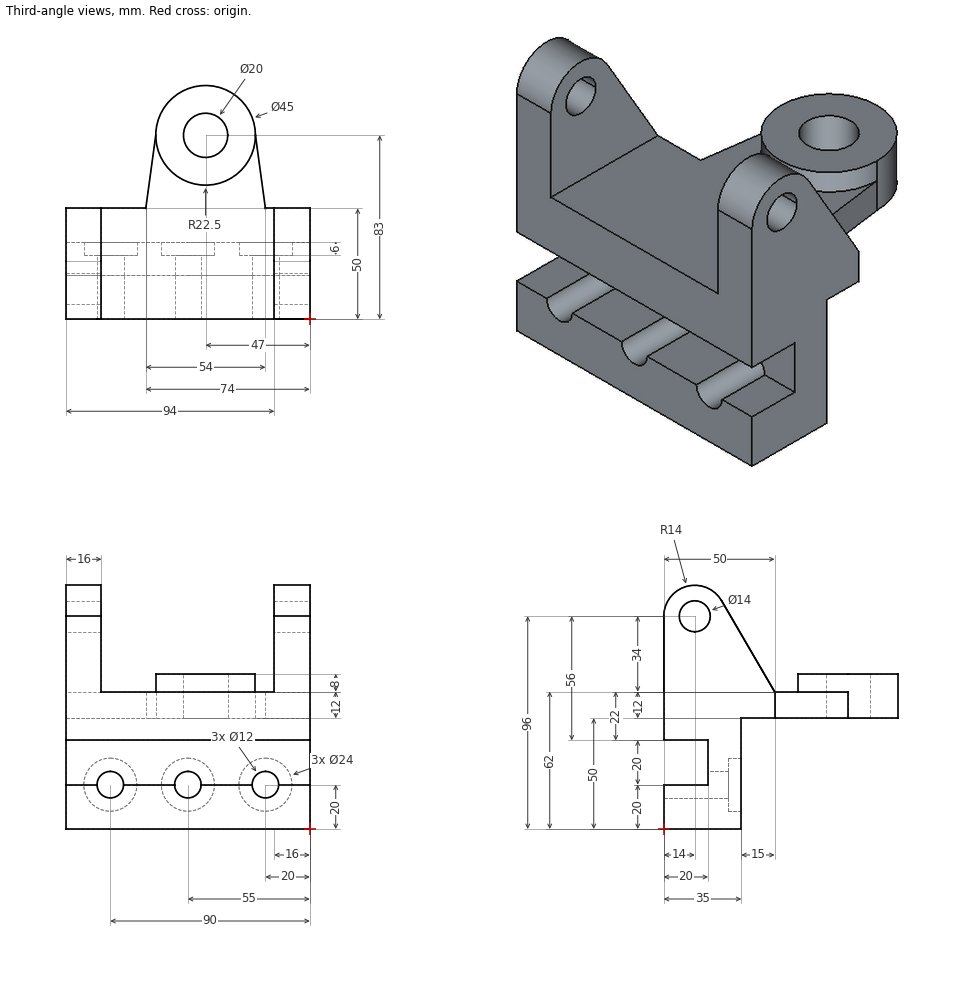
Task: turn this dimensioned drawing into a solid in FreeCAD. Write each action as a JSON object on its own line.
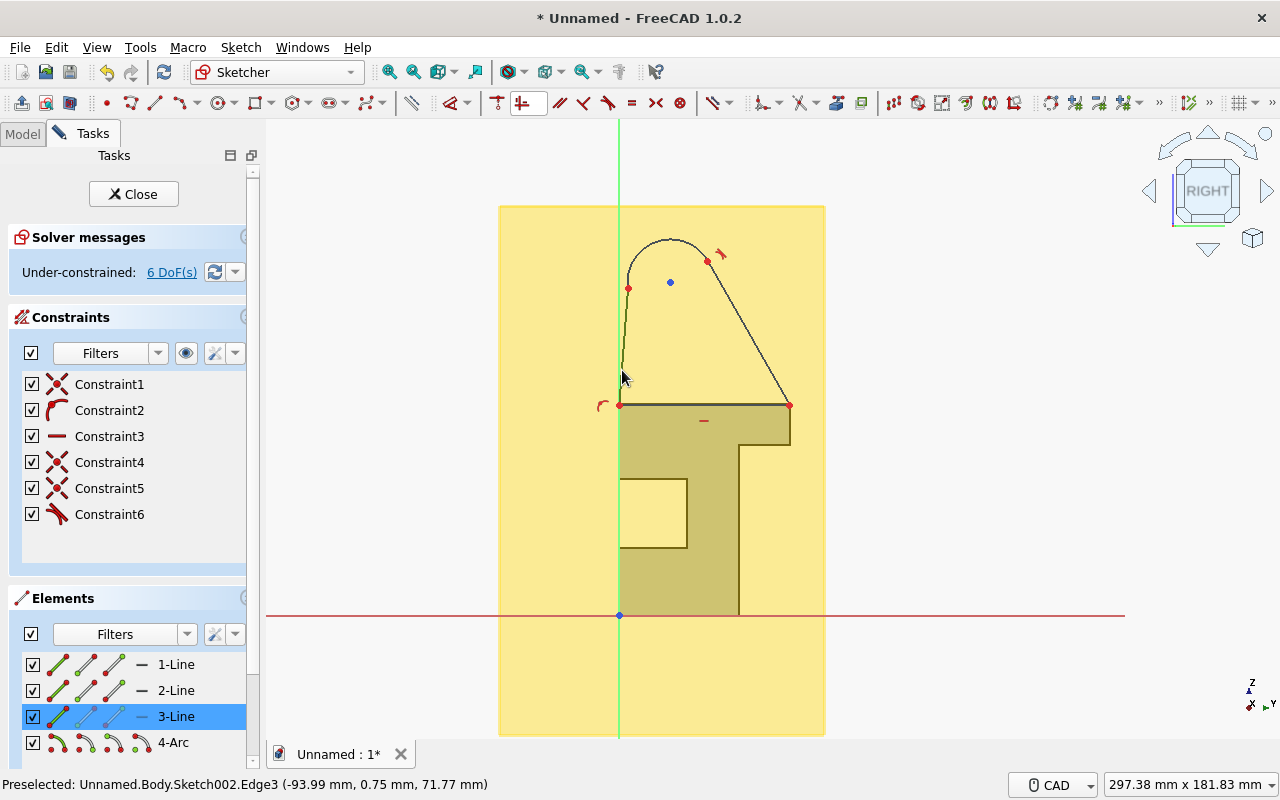
{"action": "left_click", "coordinate": [680, 241]}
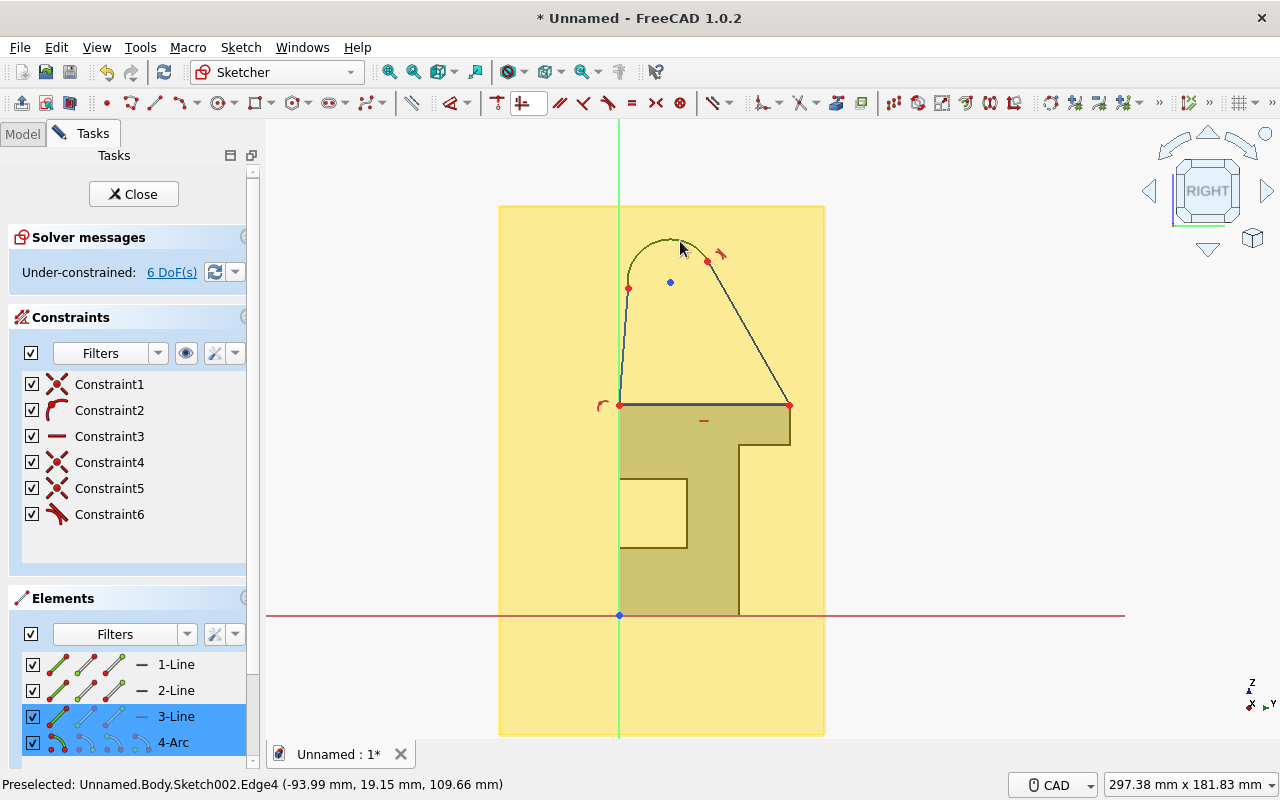
{"action": "left_click", "coordinate": [608, 104]}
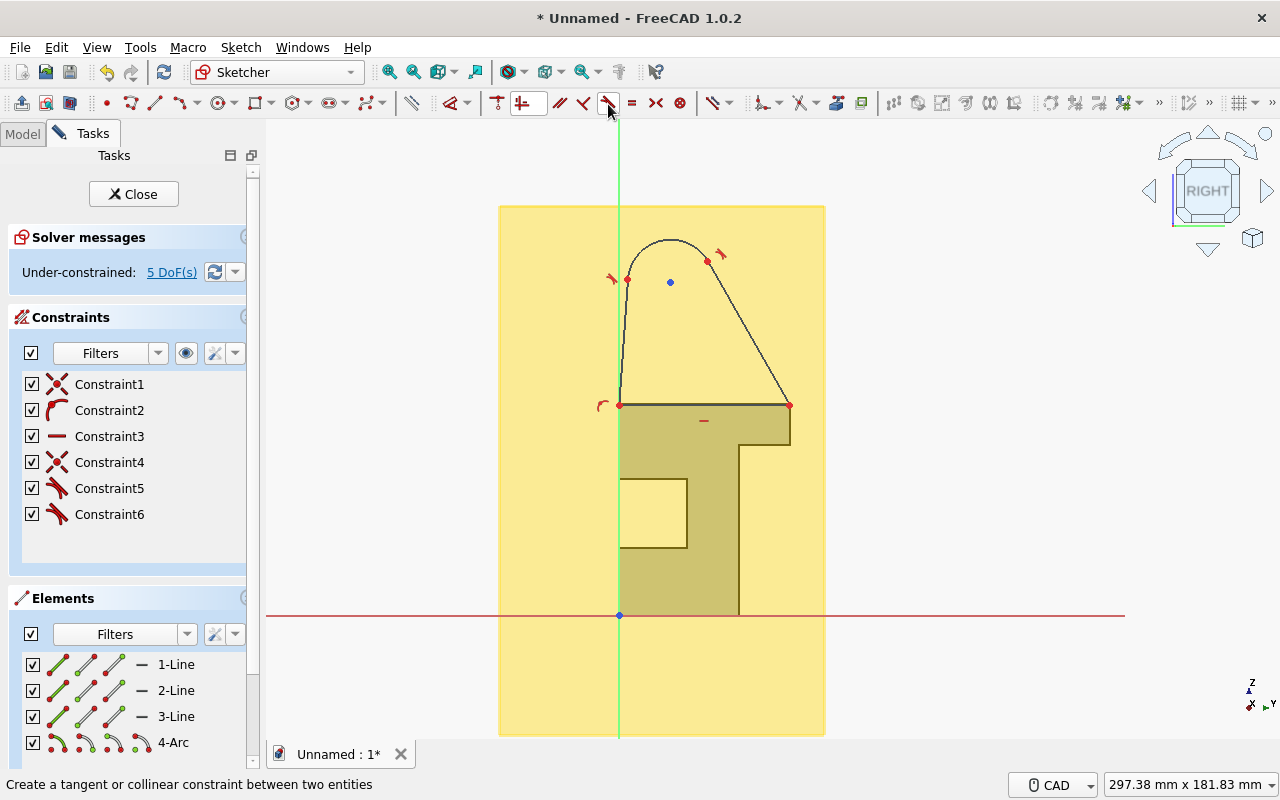
{"action": "left_click", "coordinate": [622, 367]}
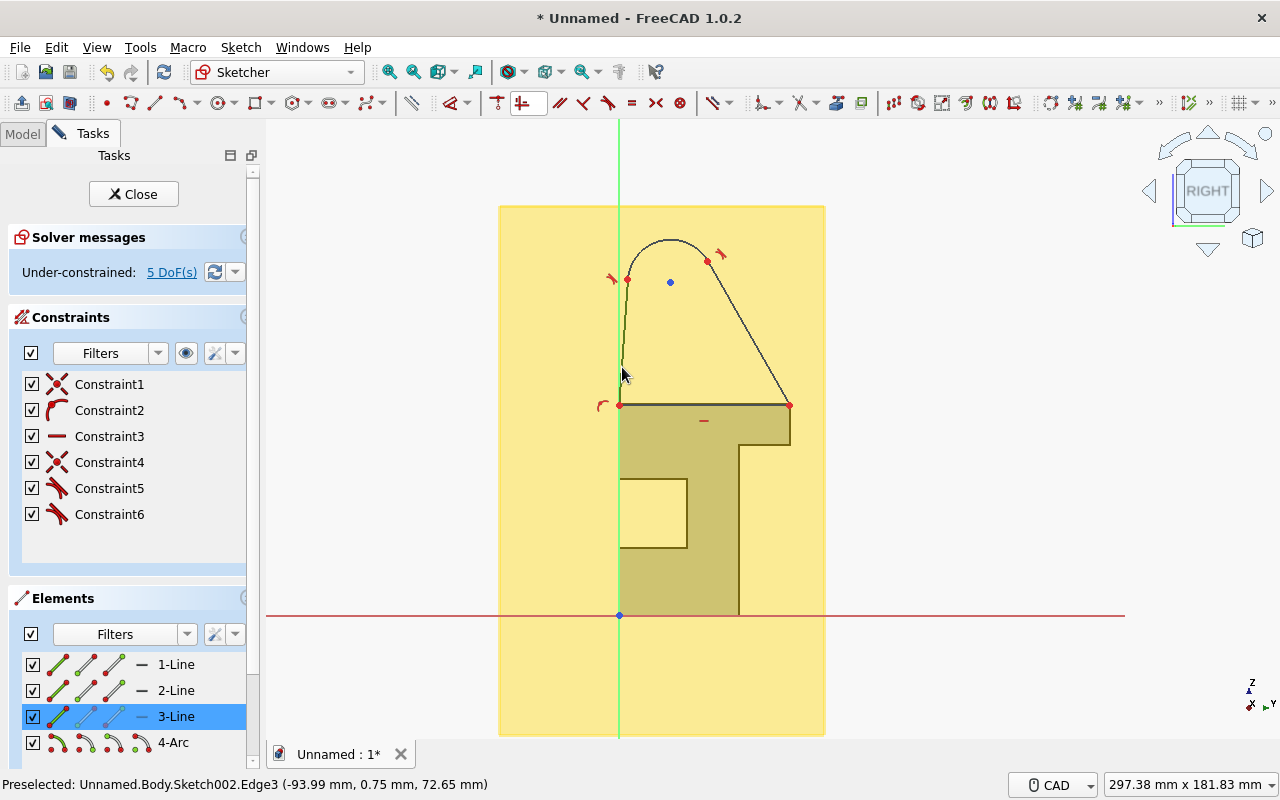
{"action": "left_click", "coordinate": [542, 104]}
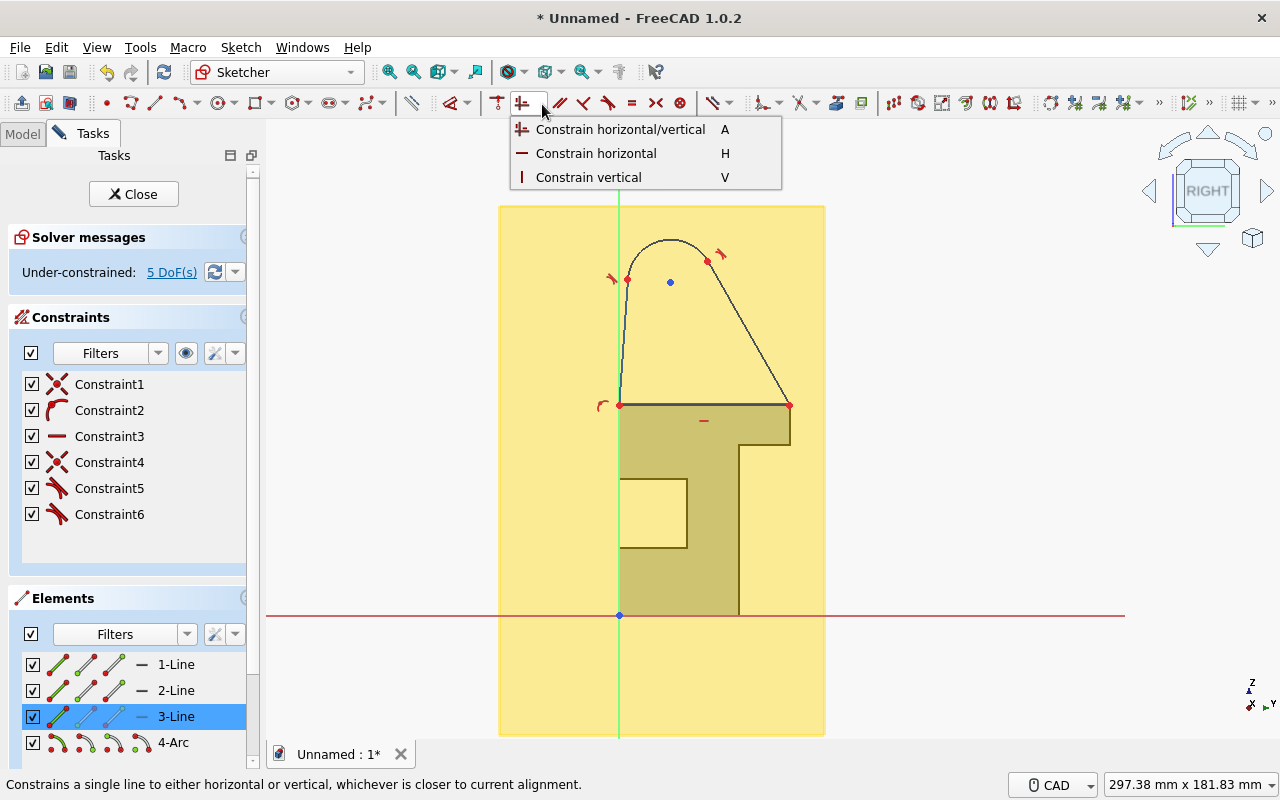
{"action": "left_click", "coordinate": [646, 177]}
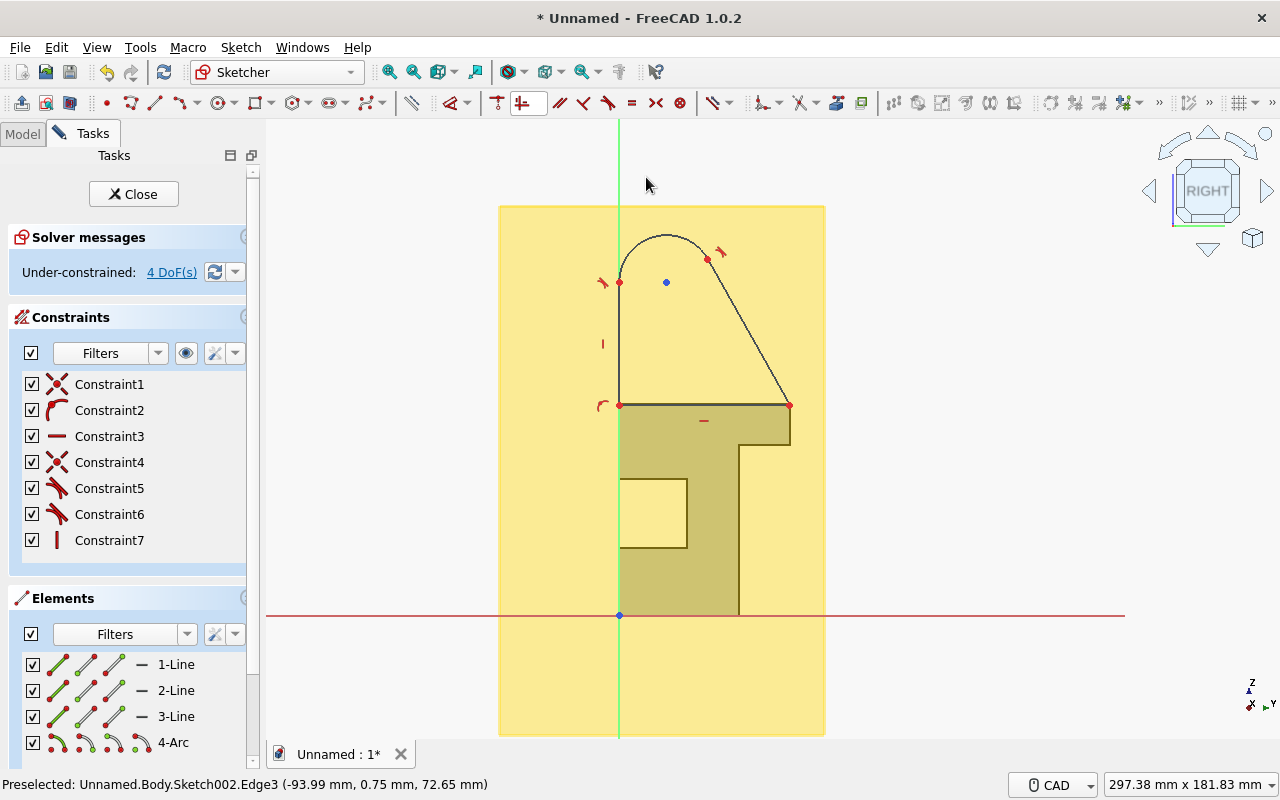
{"action": "left_click", "coordinate": [450, 104]}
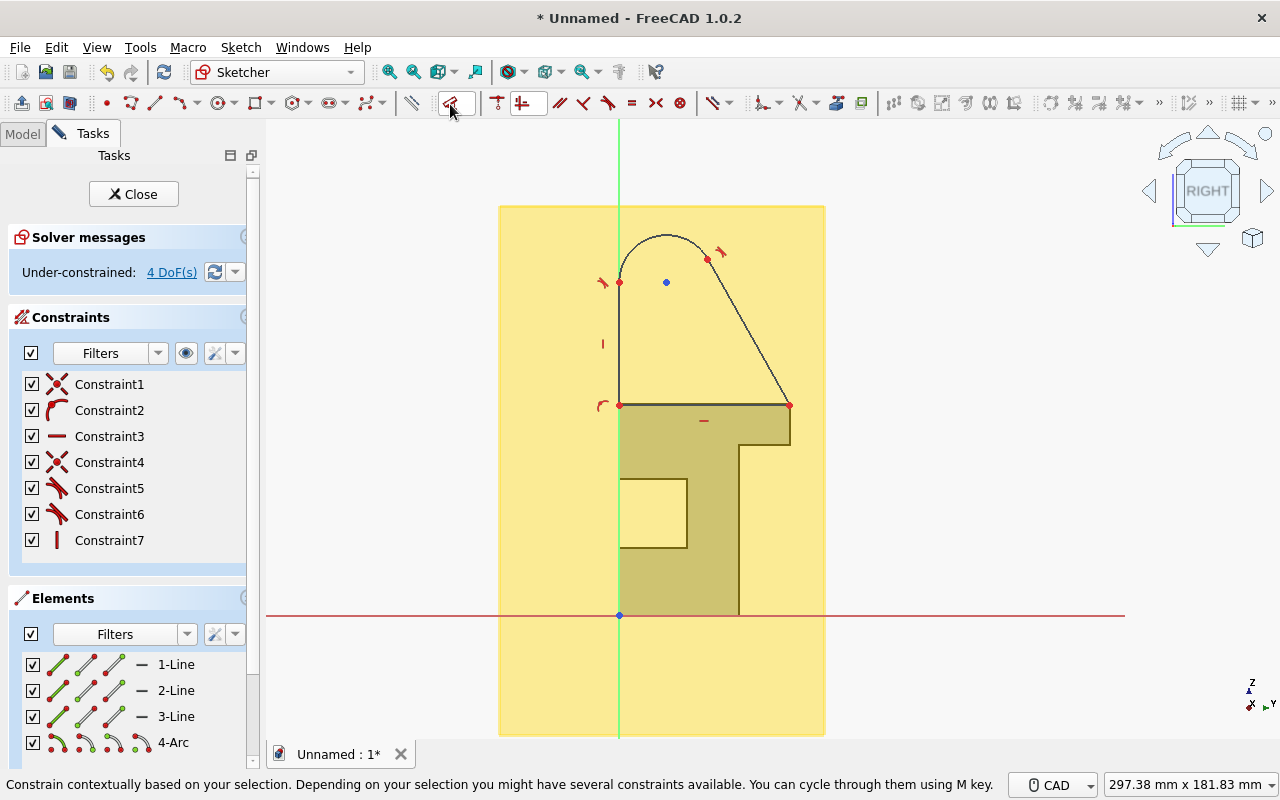
{"action": "left_click", "coordinate": [679, 237]}
{"action": "left_click", "coordinate": [687, 206]}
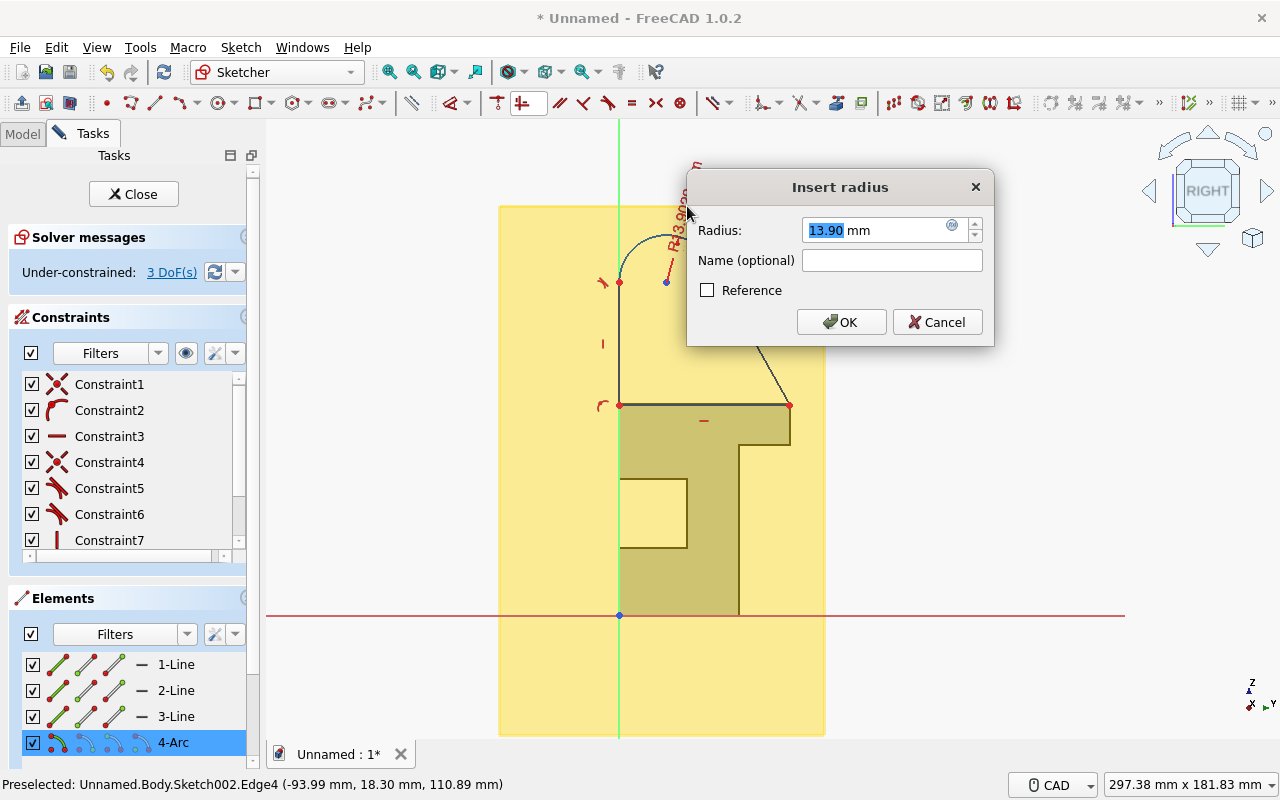
{"action": "type", "text": "14"}
{"action": "key", "text": "Return"}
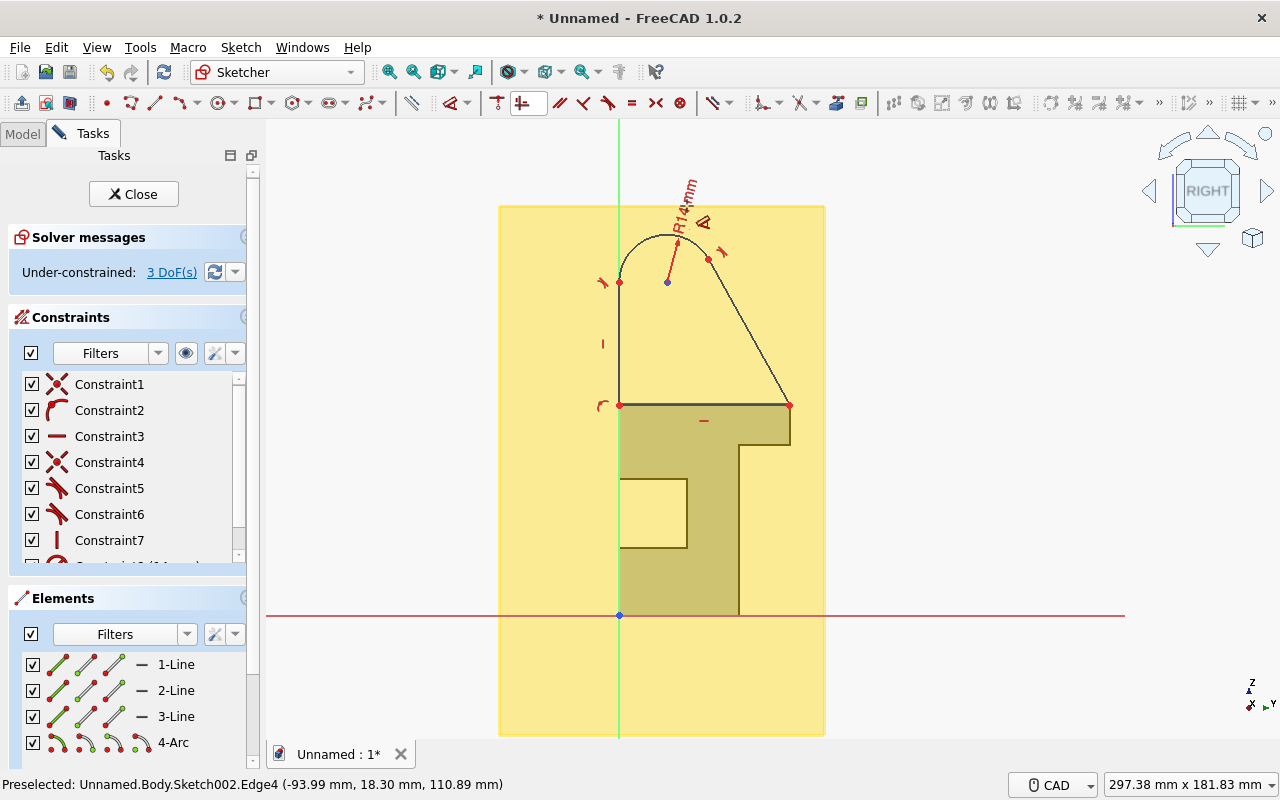
{"action": "left_click", "coordinate": [739, 405]}
{"action": "left_click", "coordinate": [705, 371]}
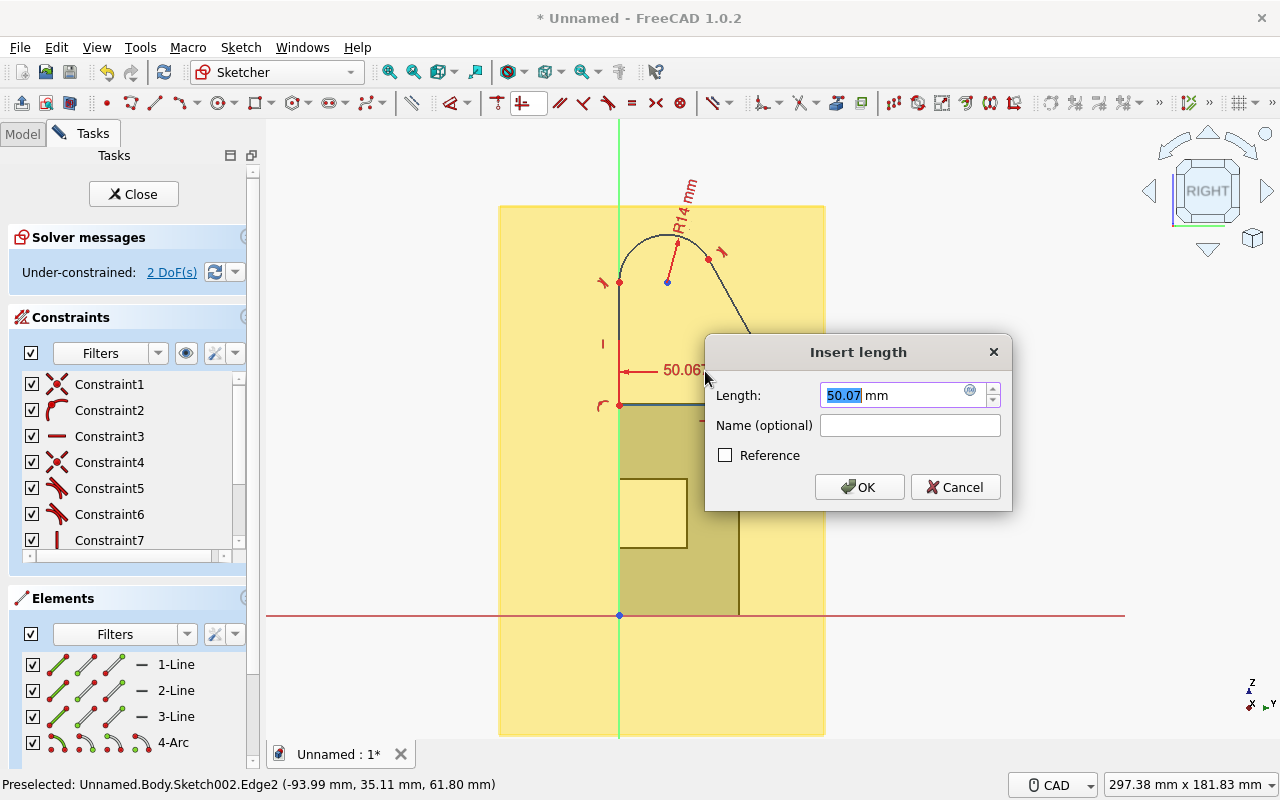
{"action": "type", "text": "50"}
{"action": "key", "text": "Return"}